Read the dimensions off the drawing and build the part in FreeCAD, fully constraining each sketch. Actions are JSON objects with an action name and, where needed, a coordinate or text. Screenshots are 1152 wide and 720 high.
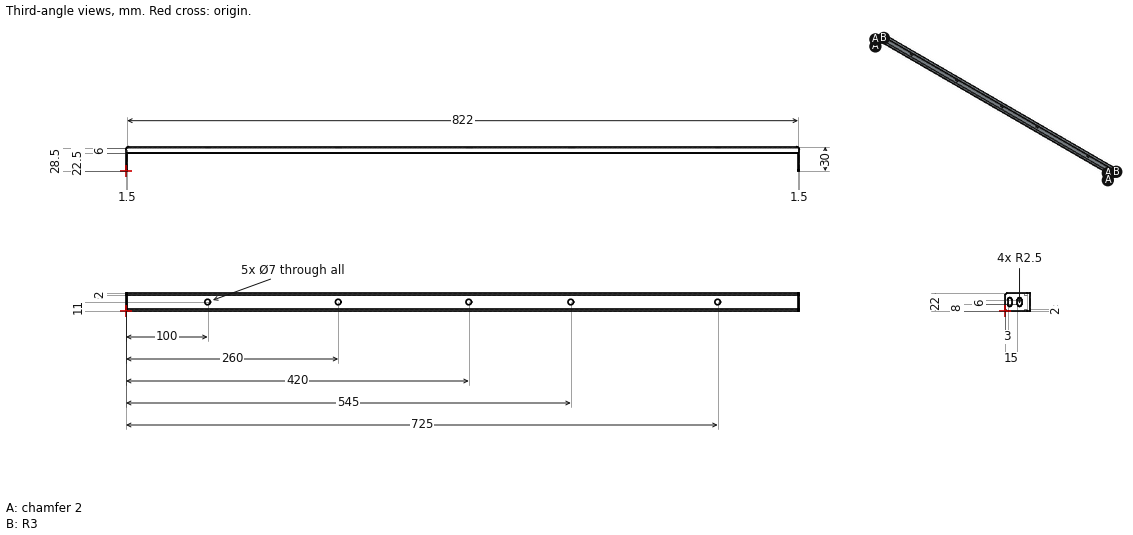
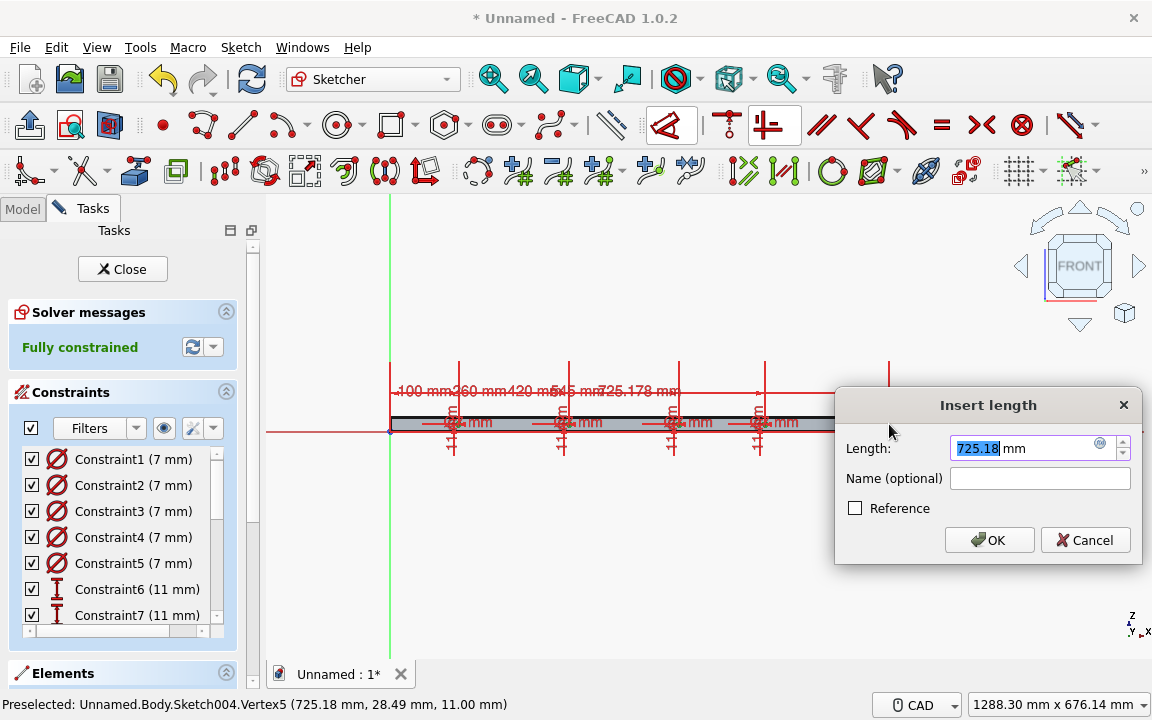
{"action": "type", "text": "725"}
{"action": "key", "text": "Return"}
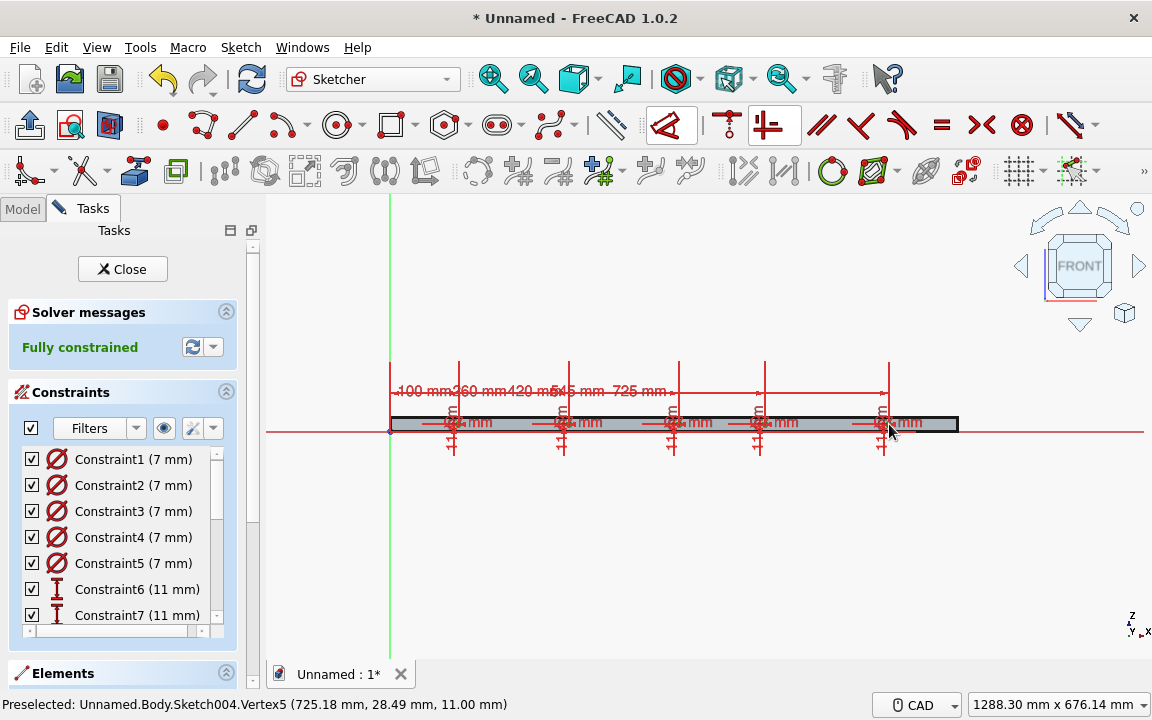
{"action": "left_click", "coordinate": [123, 269]}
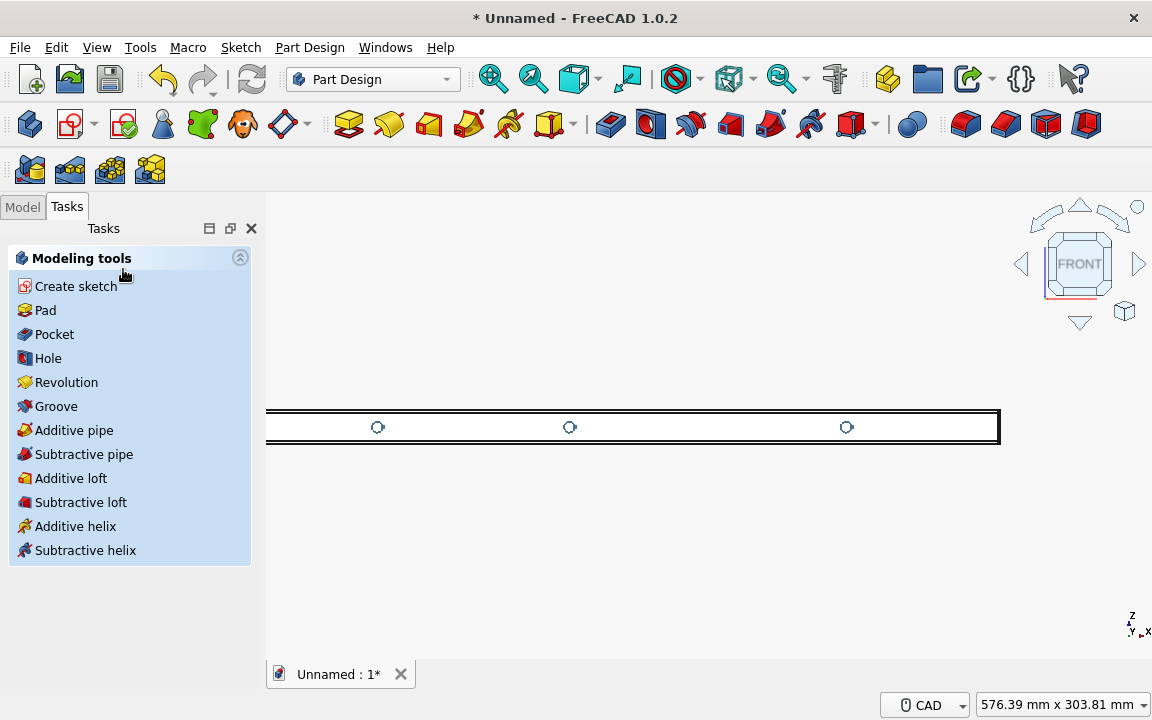
{"action": "left_click", "coordinate": [652, 124]}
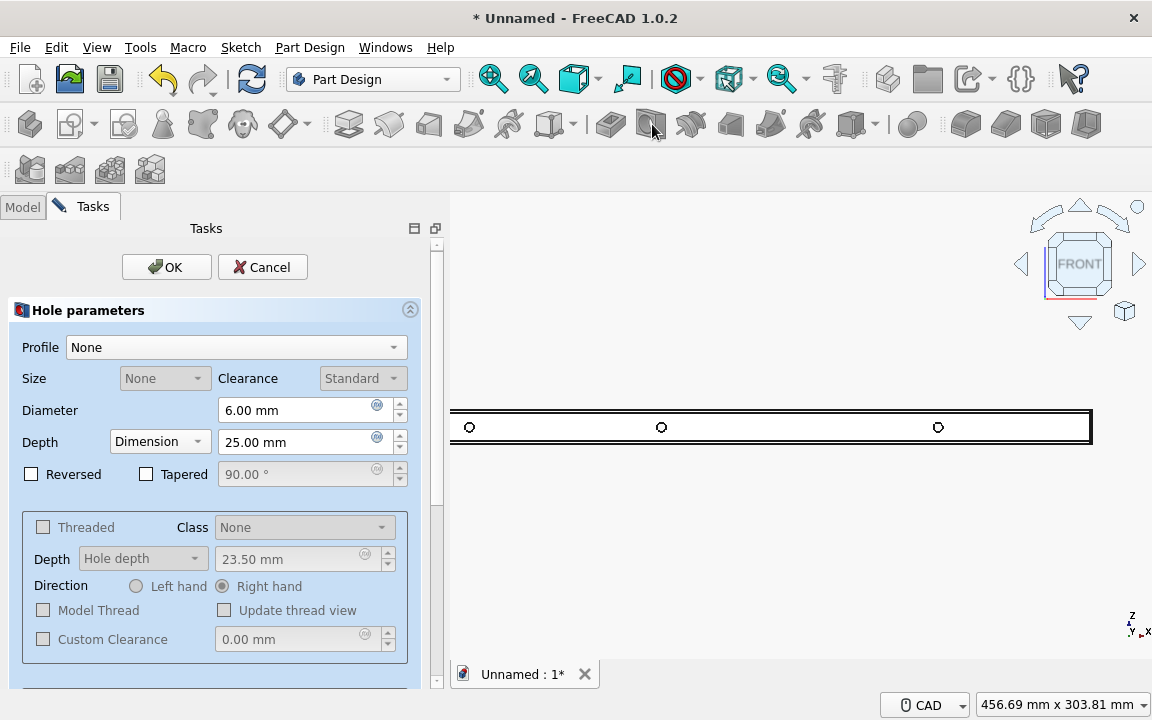
{"action": "triple_click", "coordinate": [305, 410]}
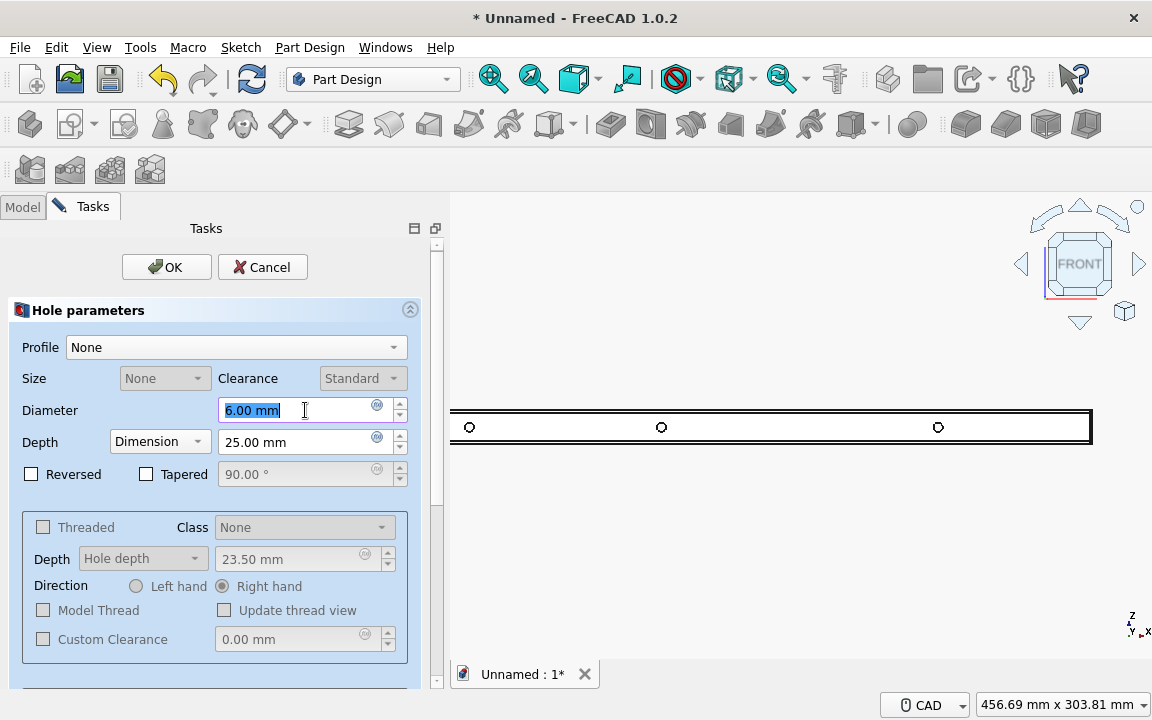
{"action": "type", "text": "7"}
{"action": "key", "text": "Tab"}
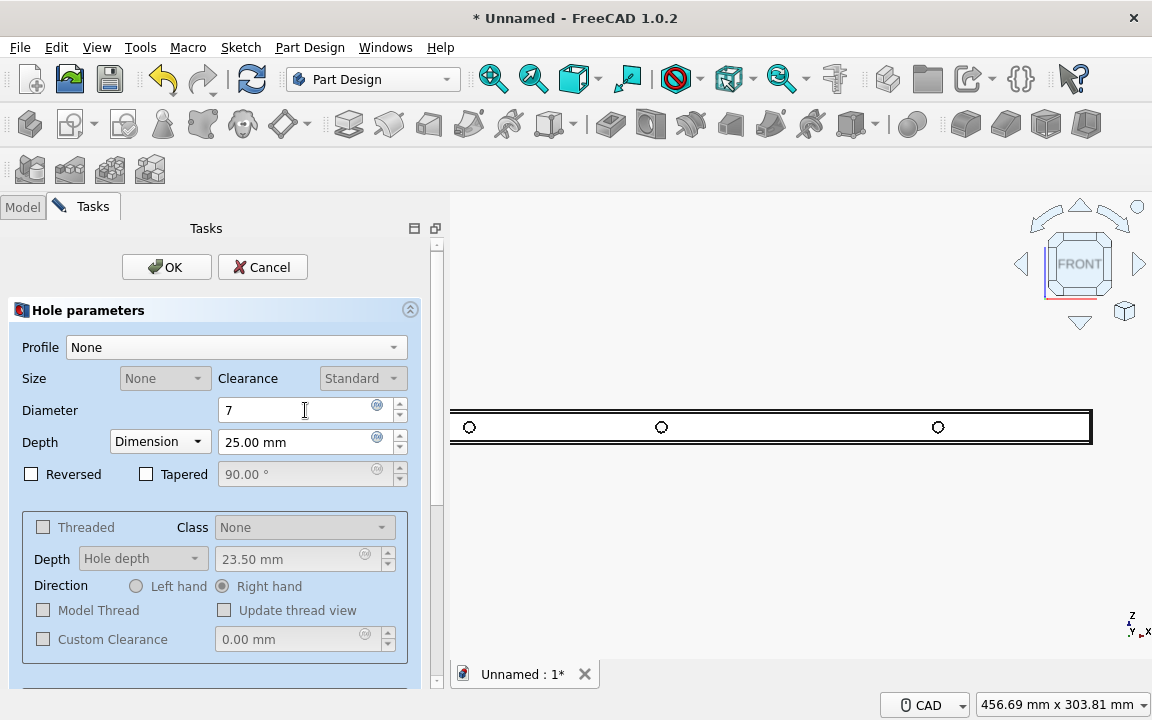
{"action": "left_click", "coordinate": [161, 442]}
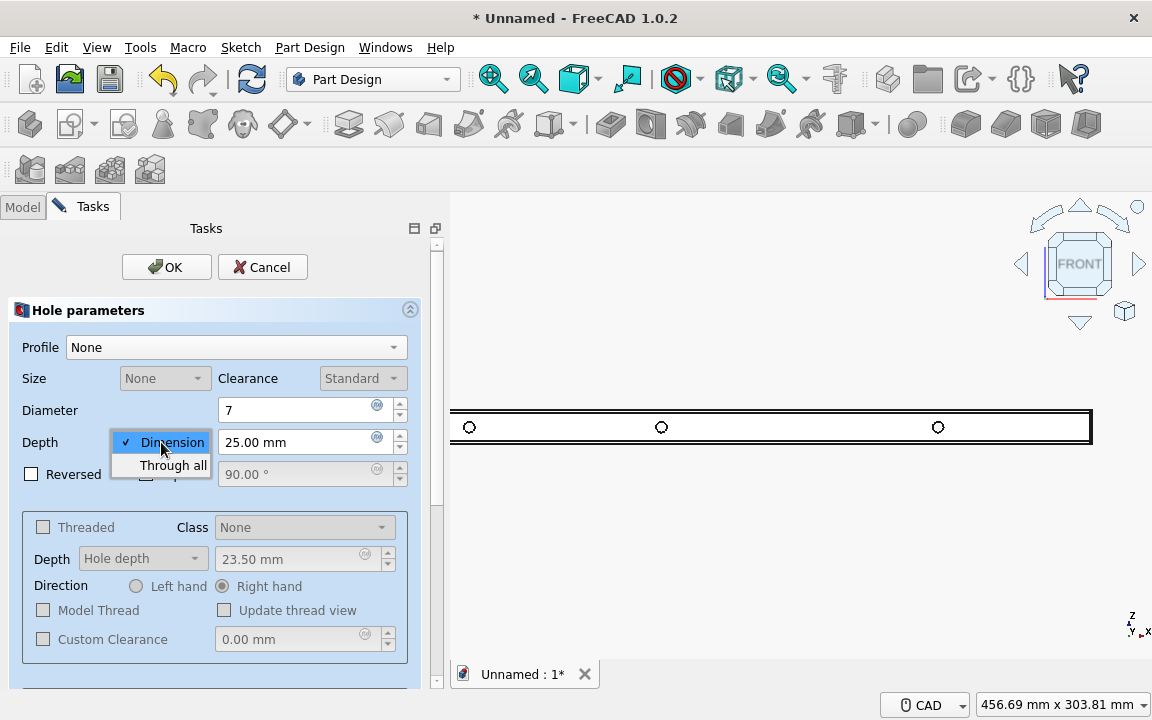
{"action": "left_click", "coordinate": [160, 466]}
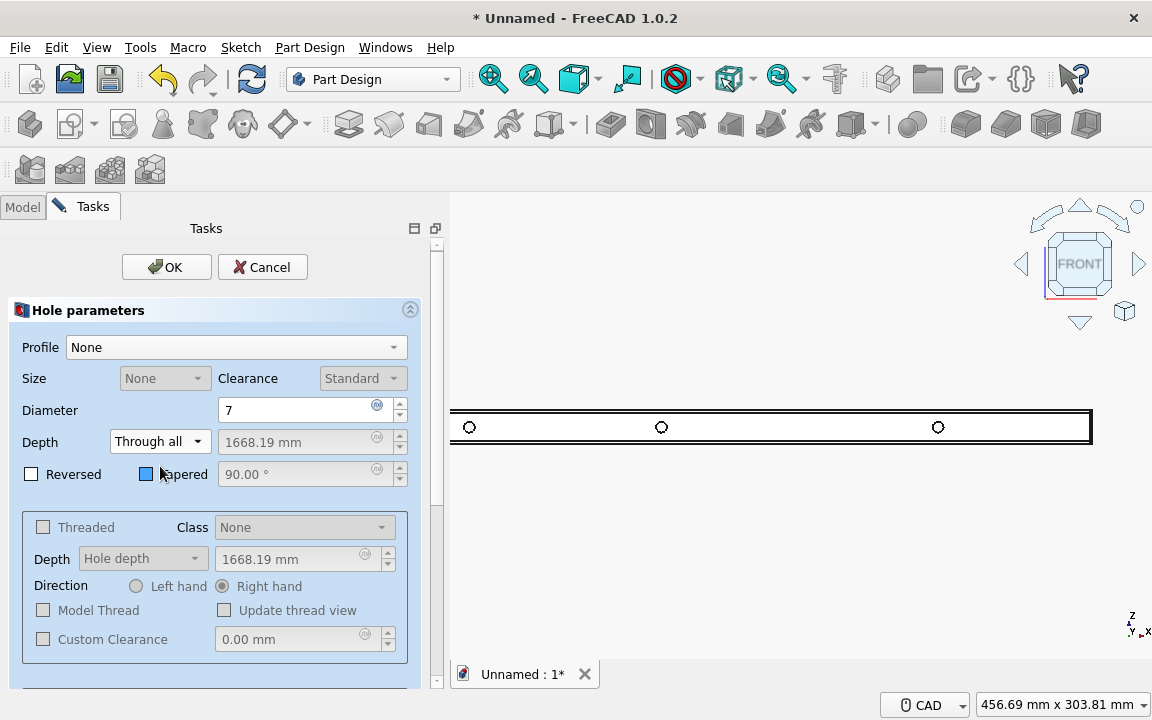
{"action": "left_click", "coordinate": [167, 267]}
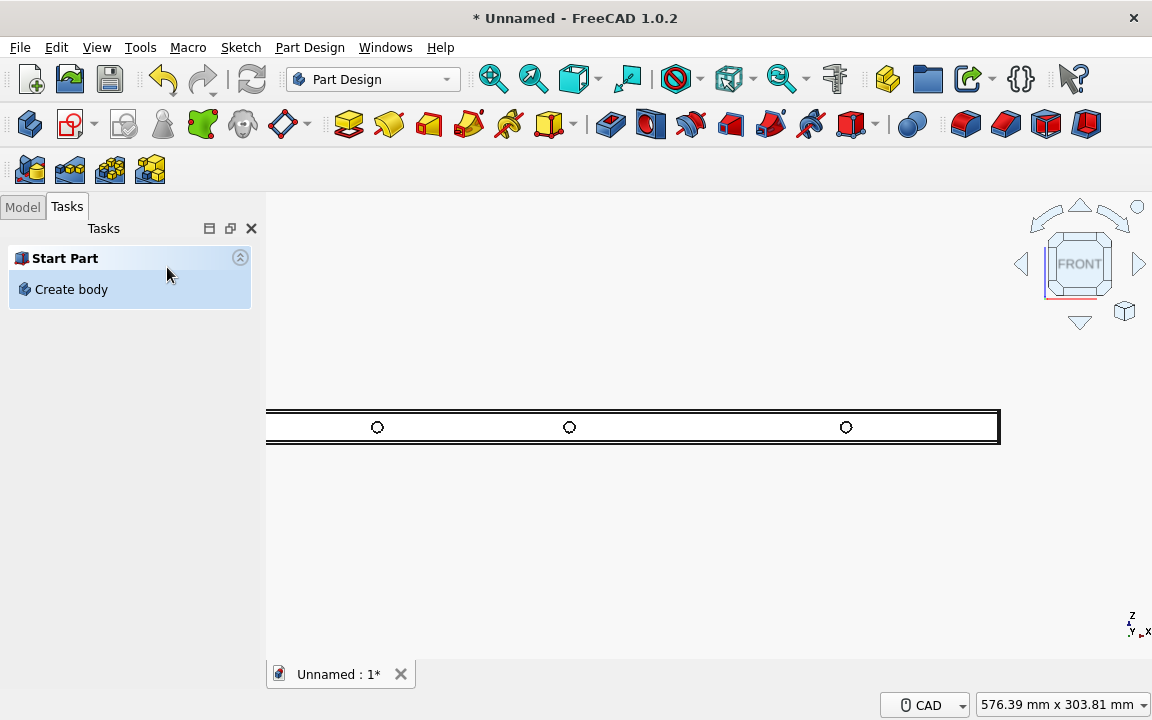
{"action": "key", "text": "0"}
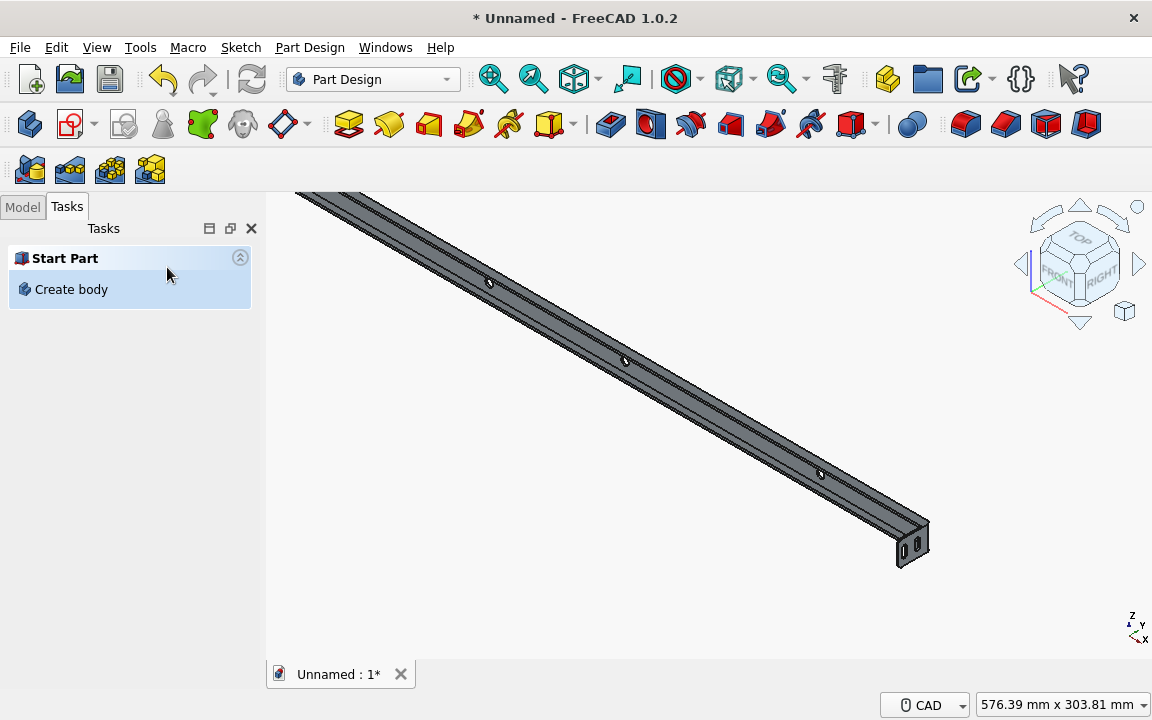
{"action": "left_click", "coordinate": [494, 80]}